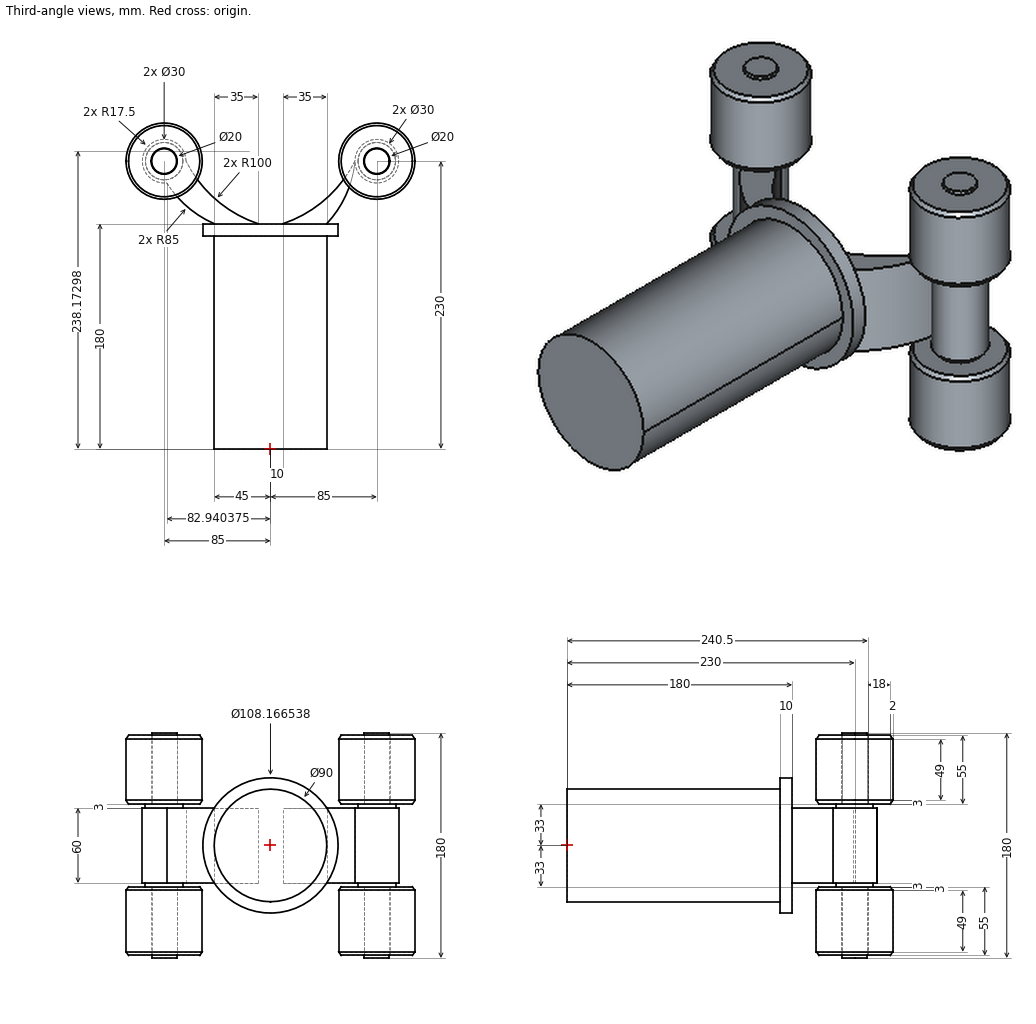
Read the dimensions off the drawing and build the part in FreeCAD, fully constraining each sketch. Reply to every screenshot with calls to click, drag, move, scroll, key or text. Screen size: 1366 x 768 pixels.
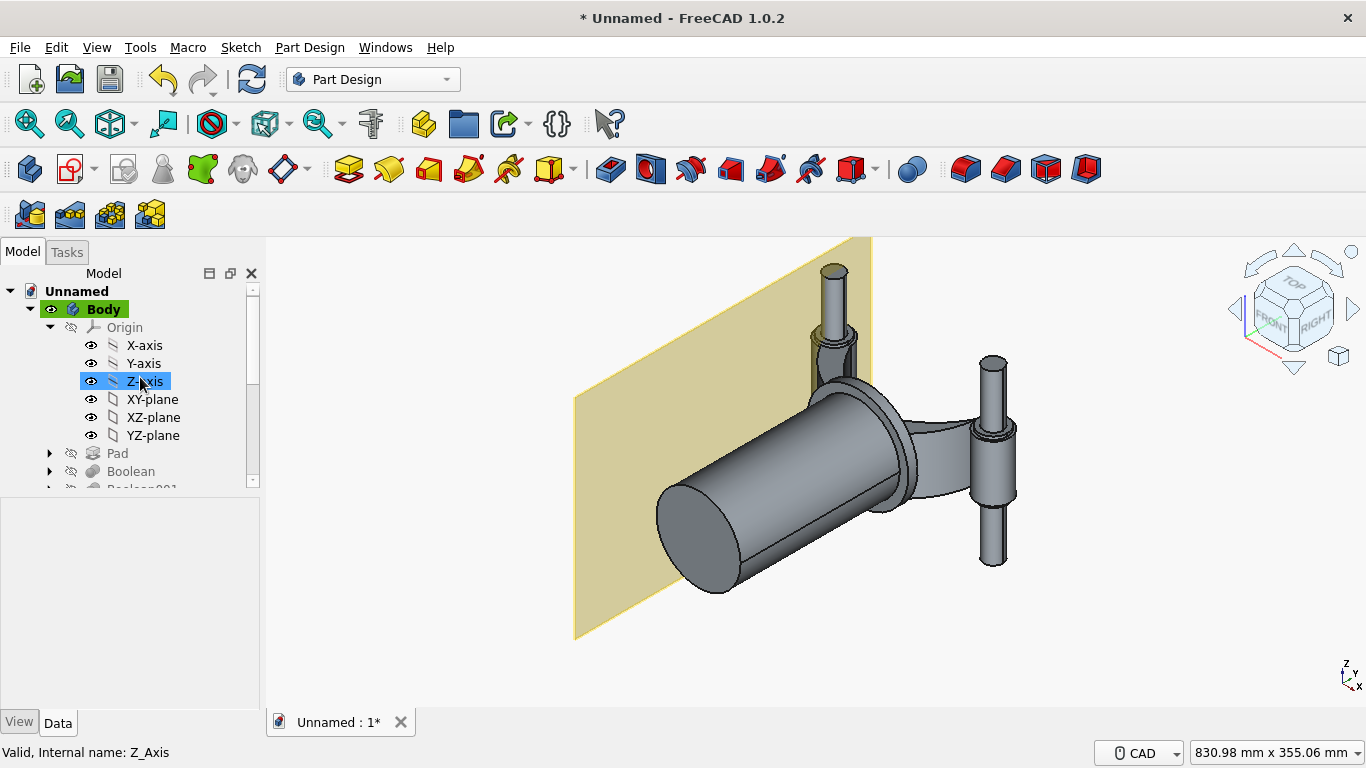
scroll(100, 377, down, 6)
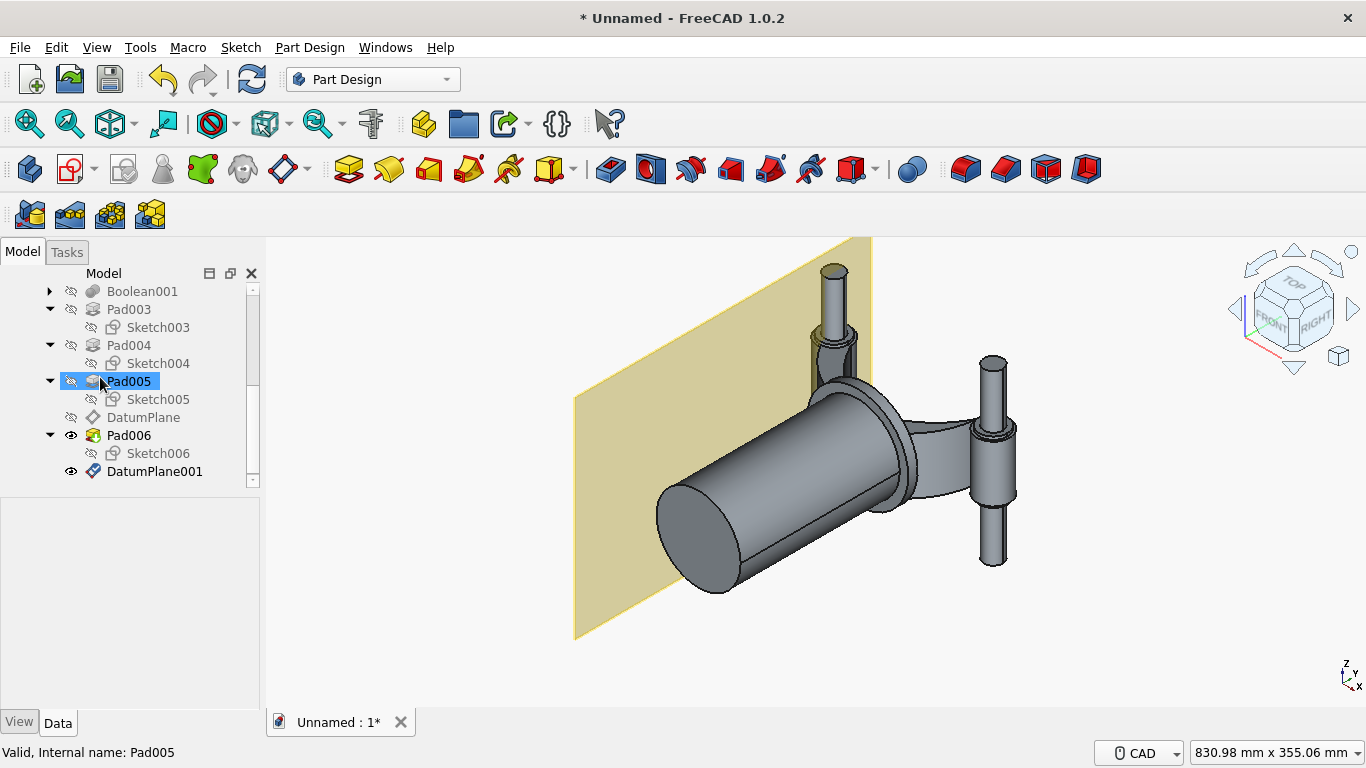
click(116, 471)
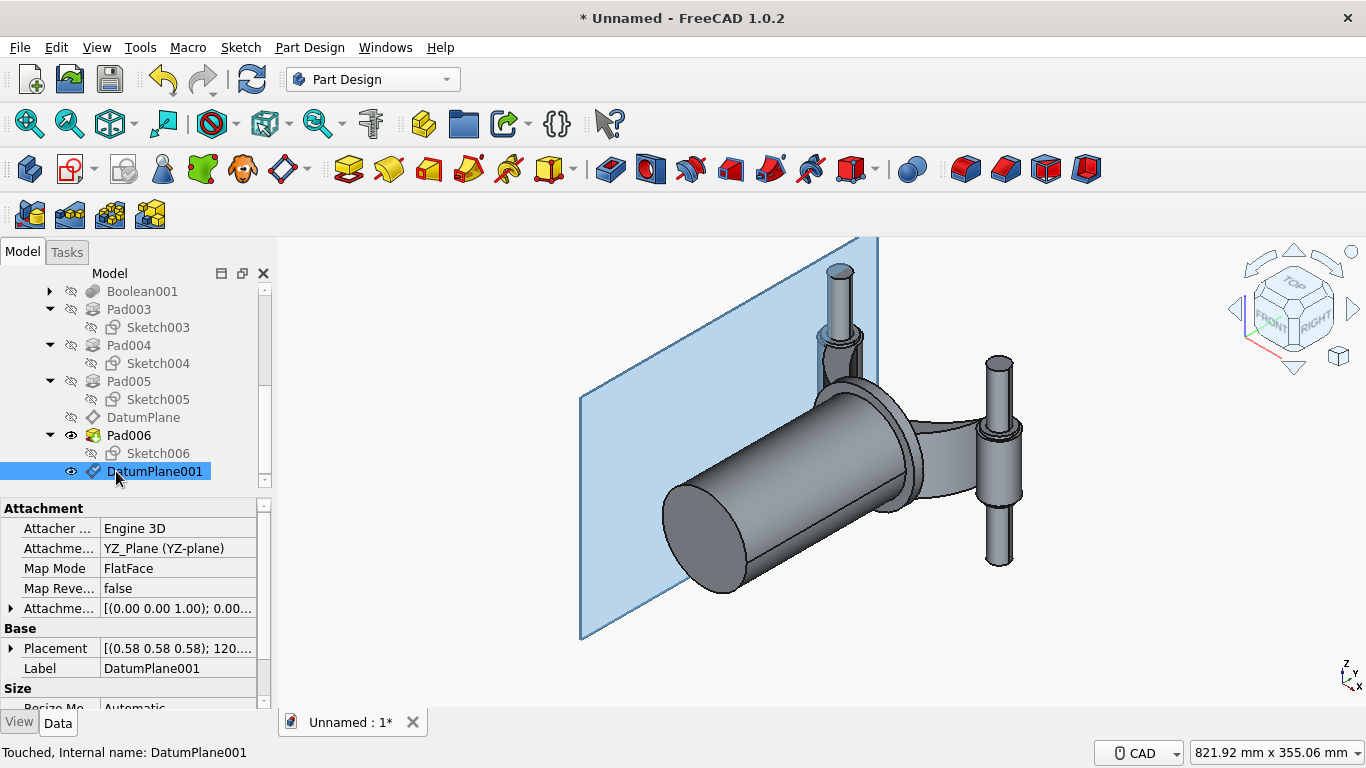
click(70, 170)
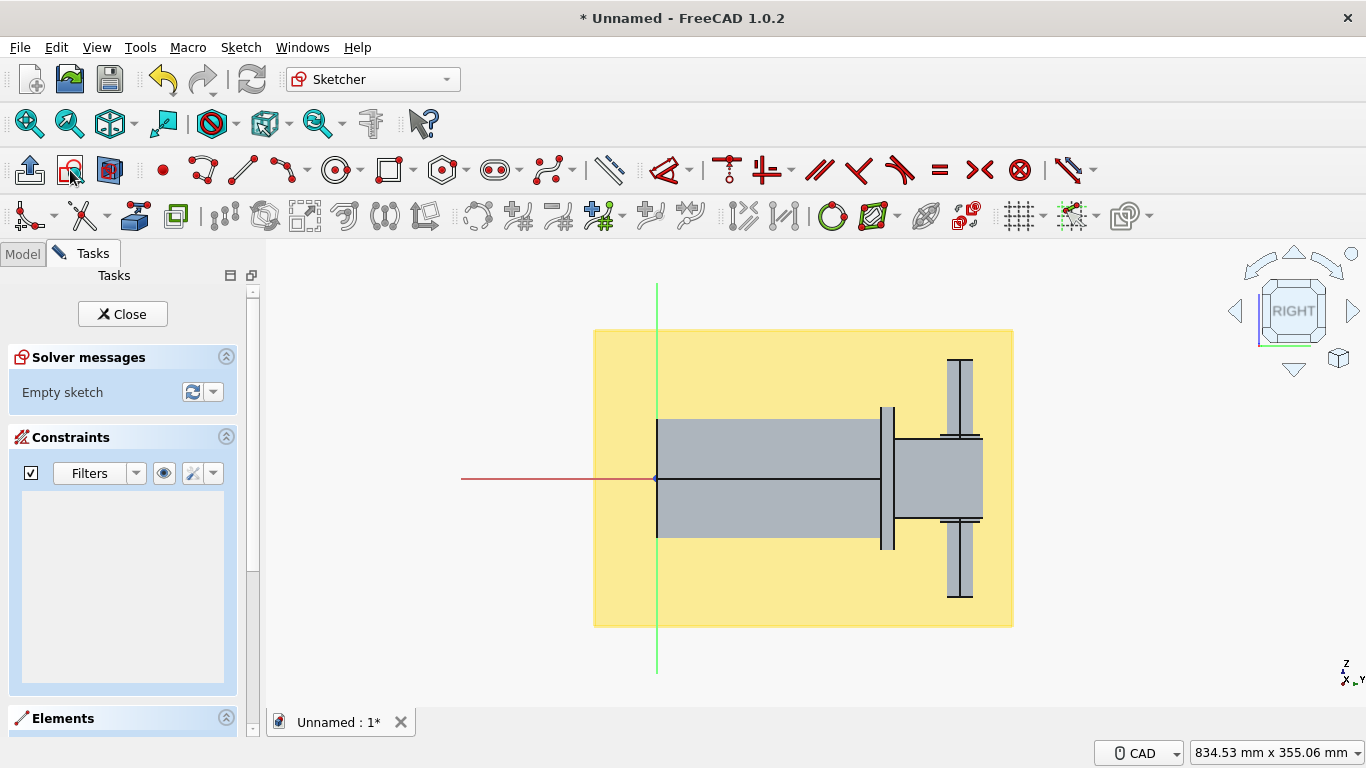
click(110, 170)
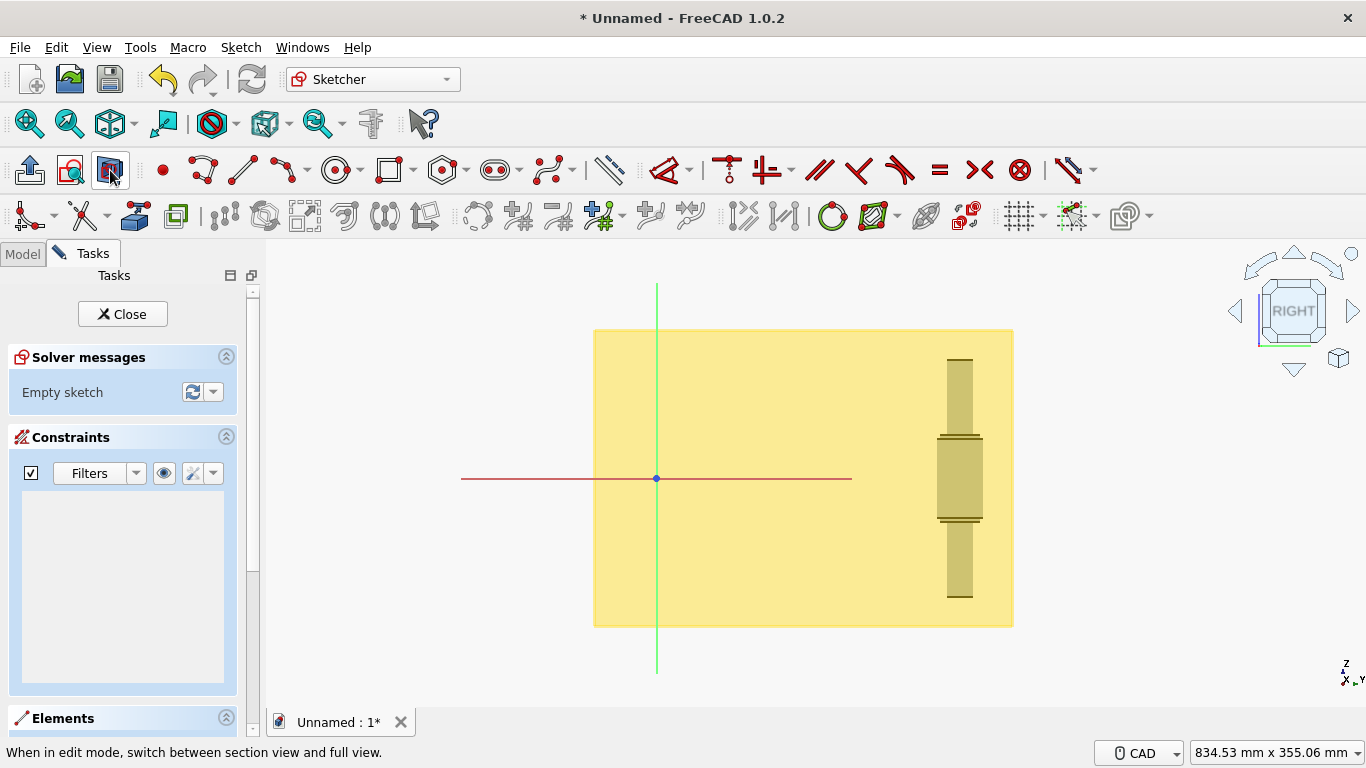
scroll(1080, 367, up, 6)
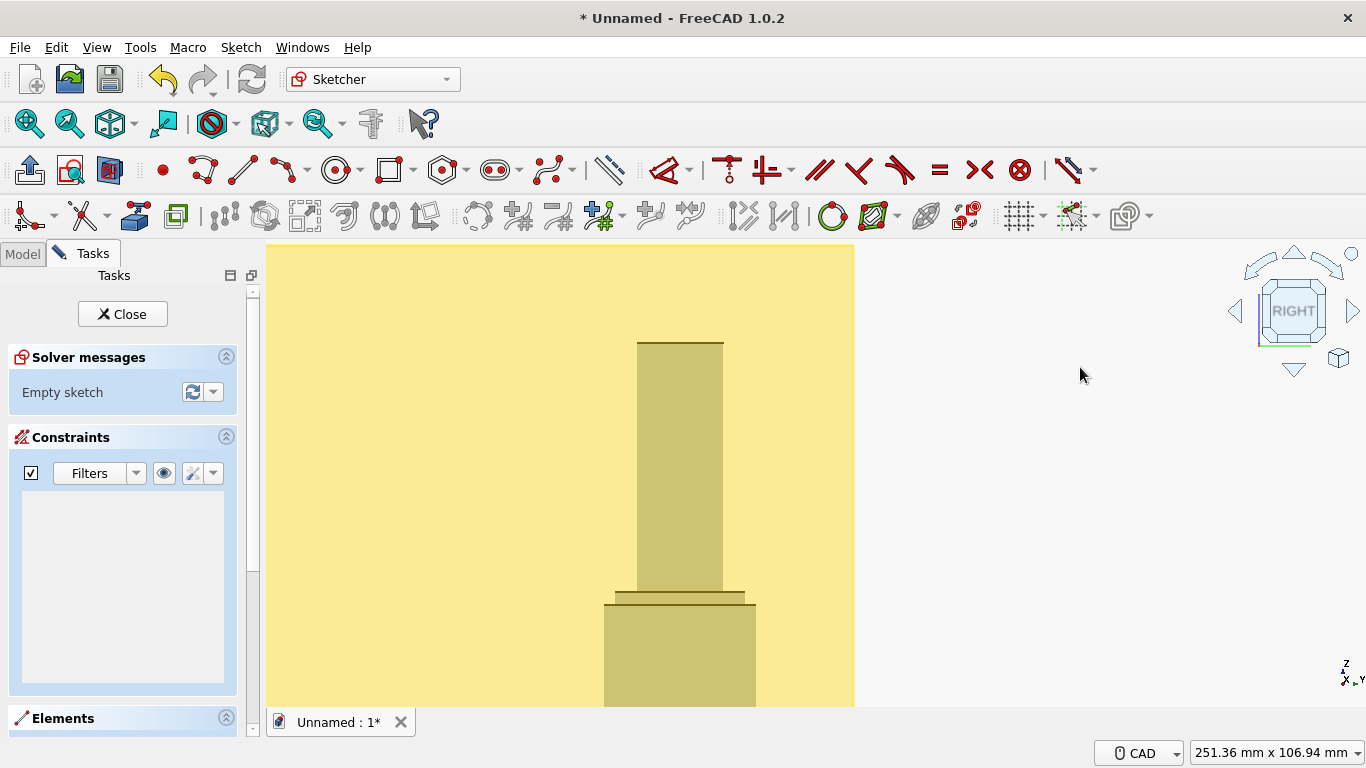
click(204, 170)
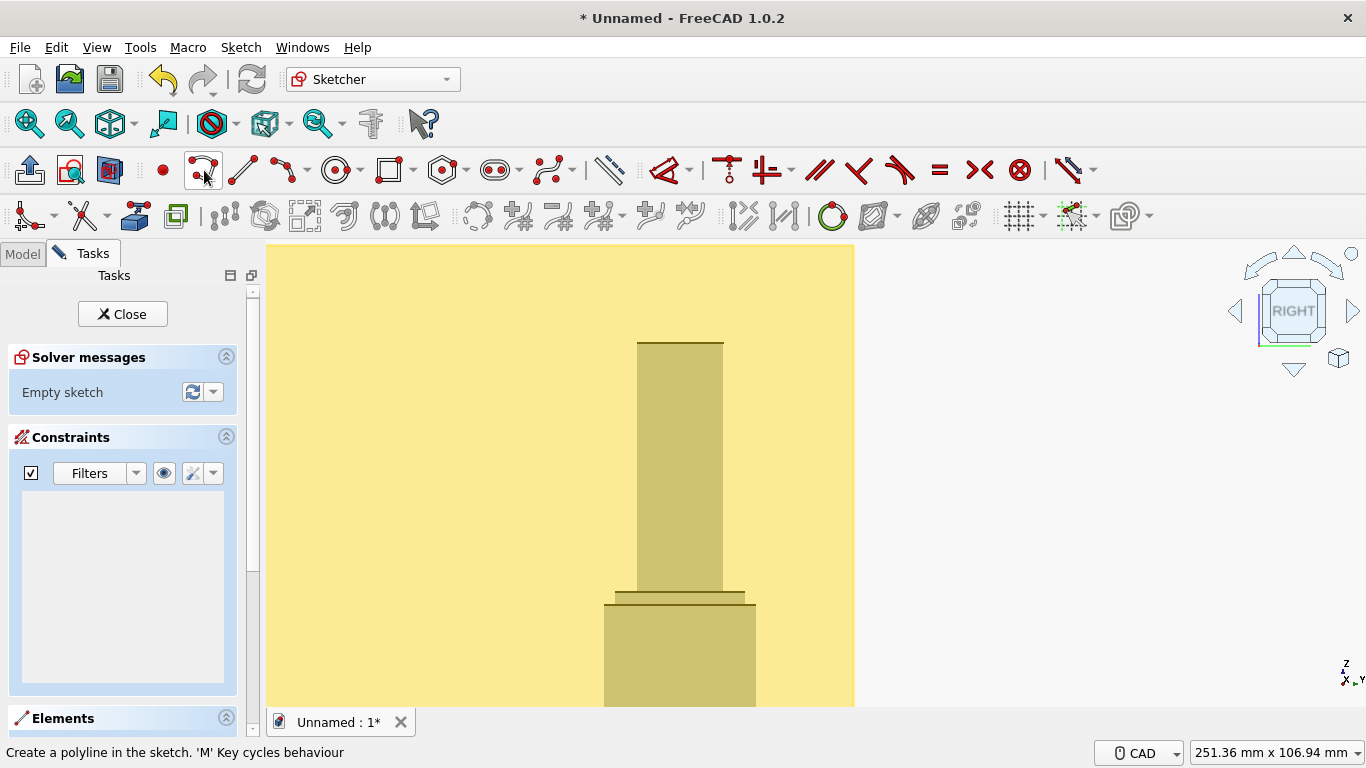
click(726, 592)
click(805, 592)
click(814, 579)
click(814, 365)
click(805, 351)
click(726, 351)
click(726, 593)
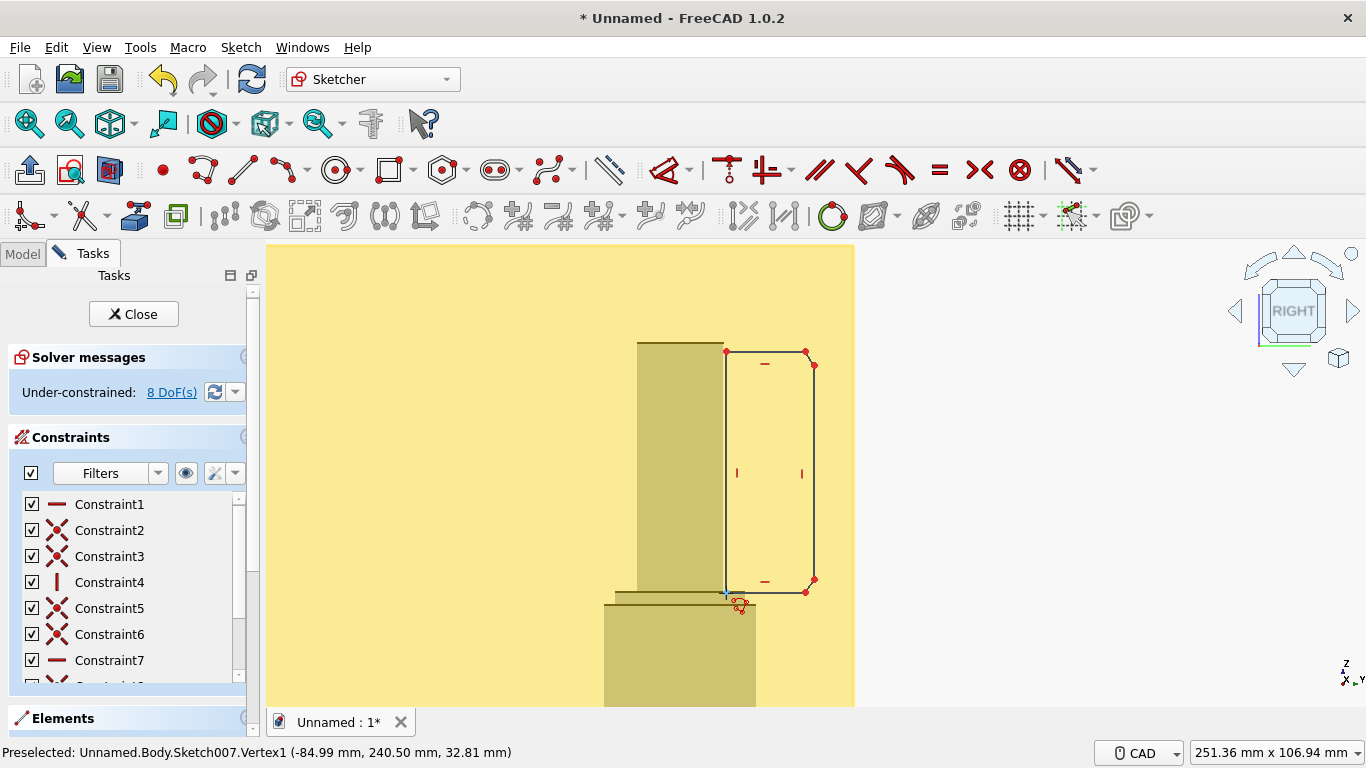
click(244, 170)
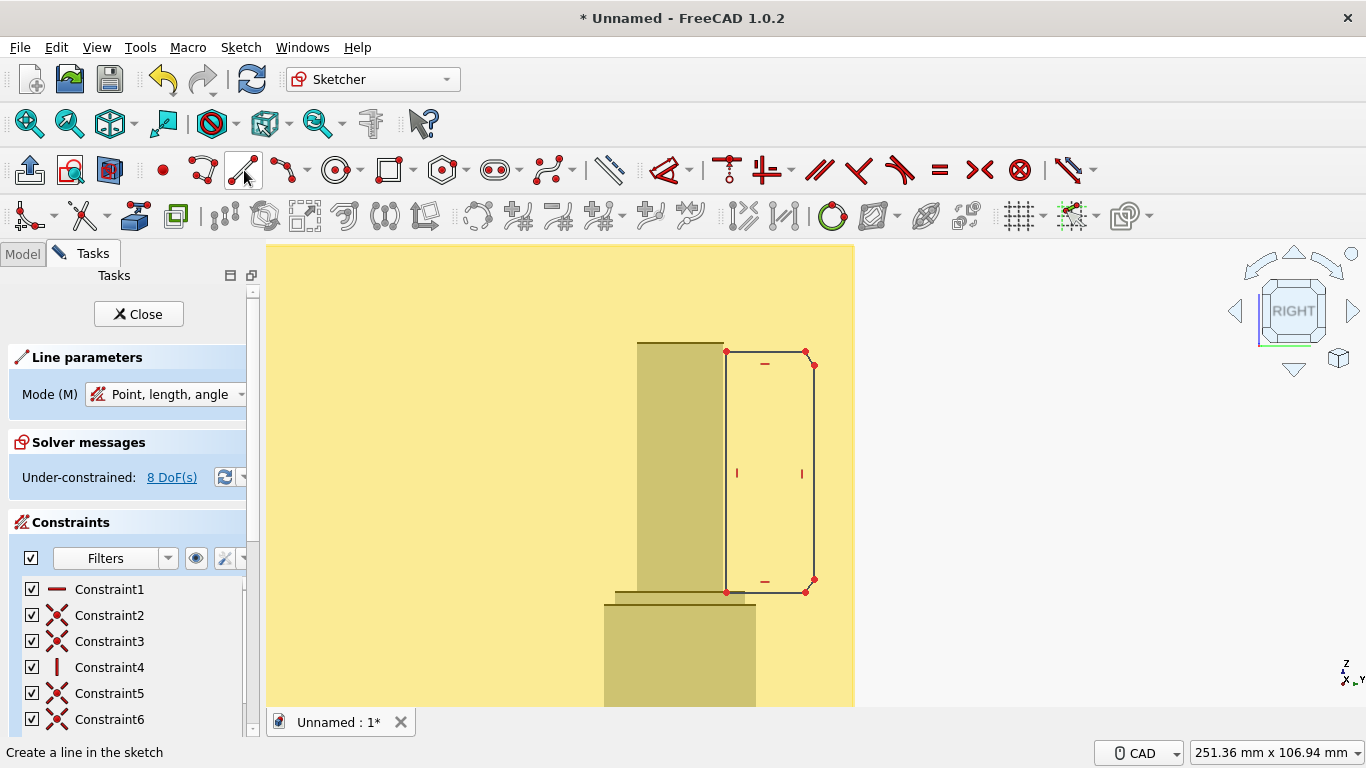
click(680, 616)
click(680, 327)
key(Escape)